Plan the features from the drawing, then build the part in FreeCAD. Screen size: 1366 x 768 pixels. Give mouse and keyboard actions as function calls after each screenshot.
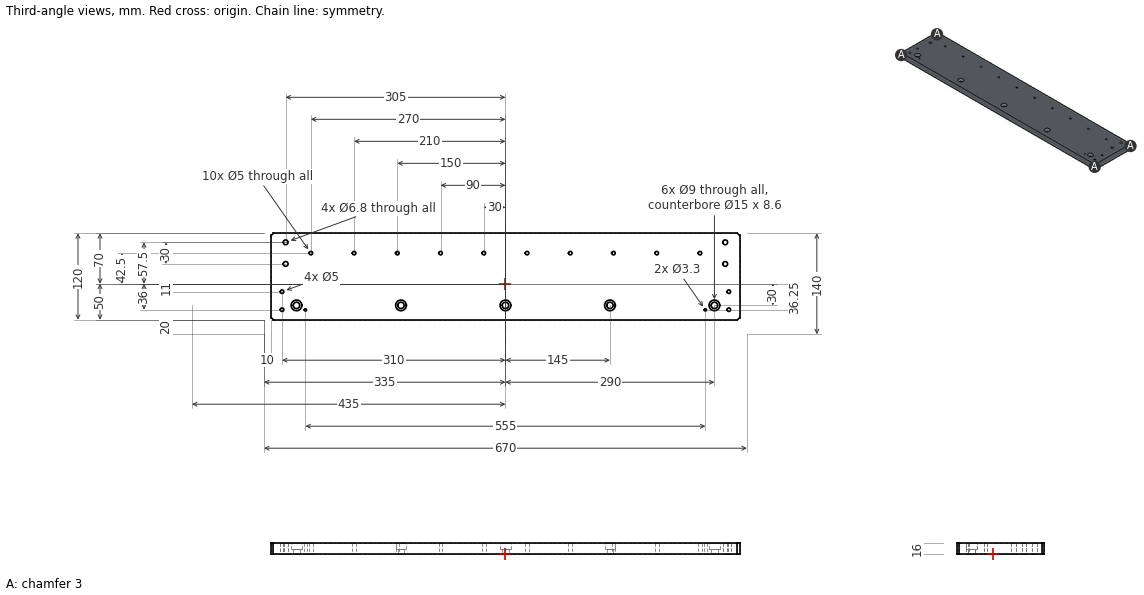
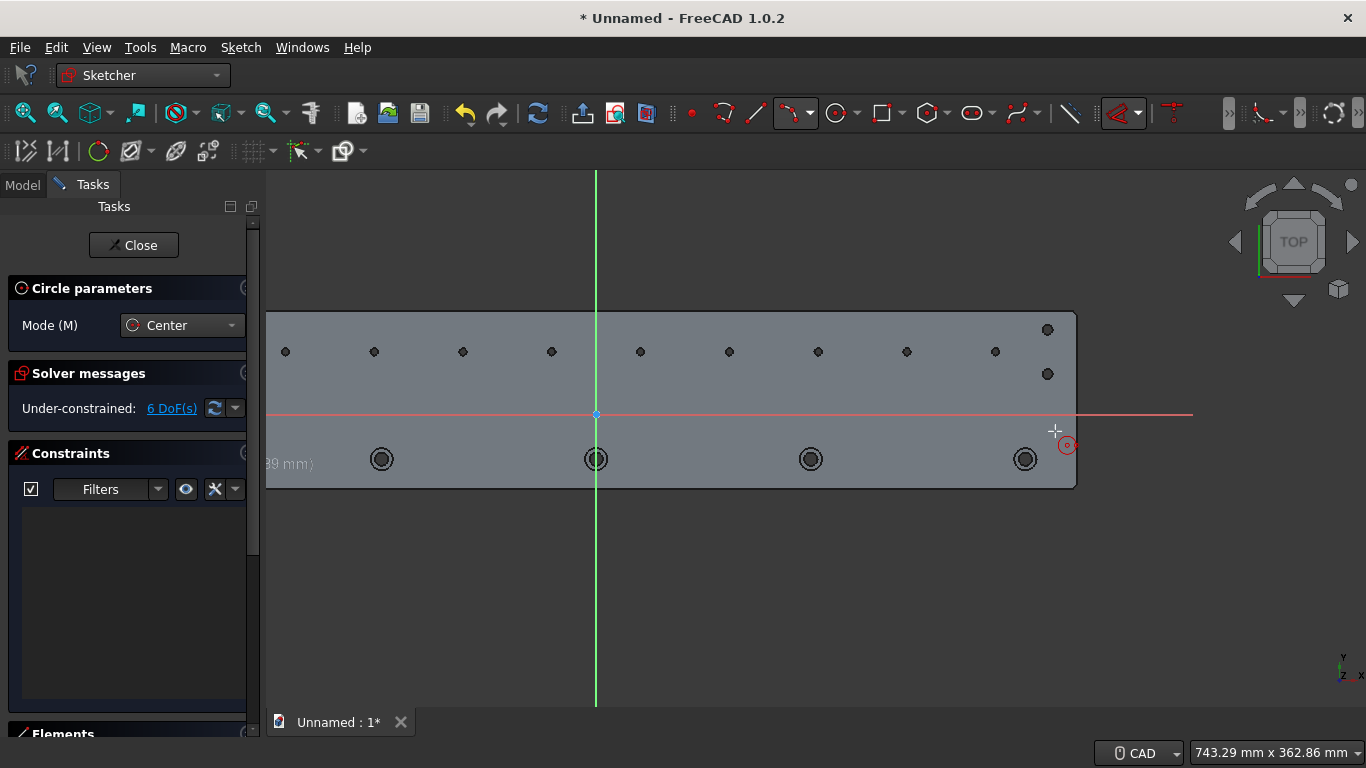
click(1055, 431)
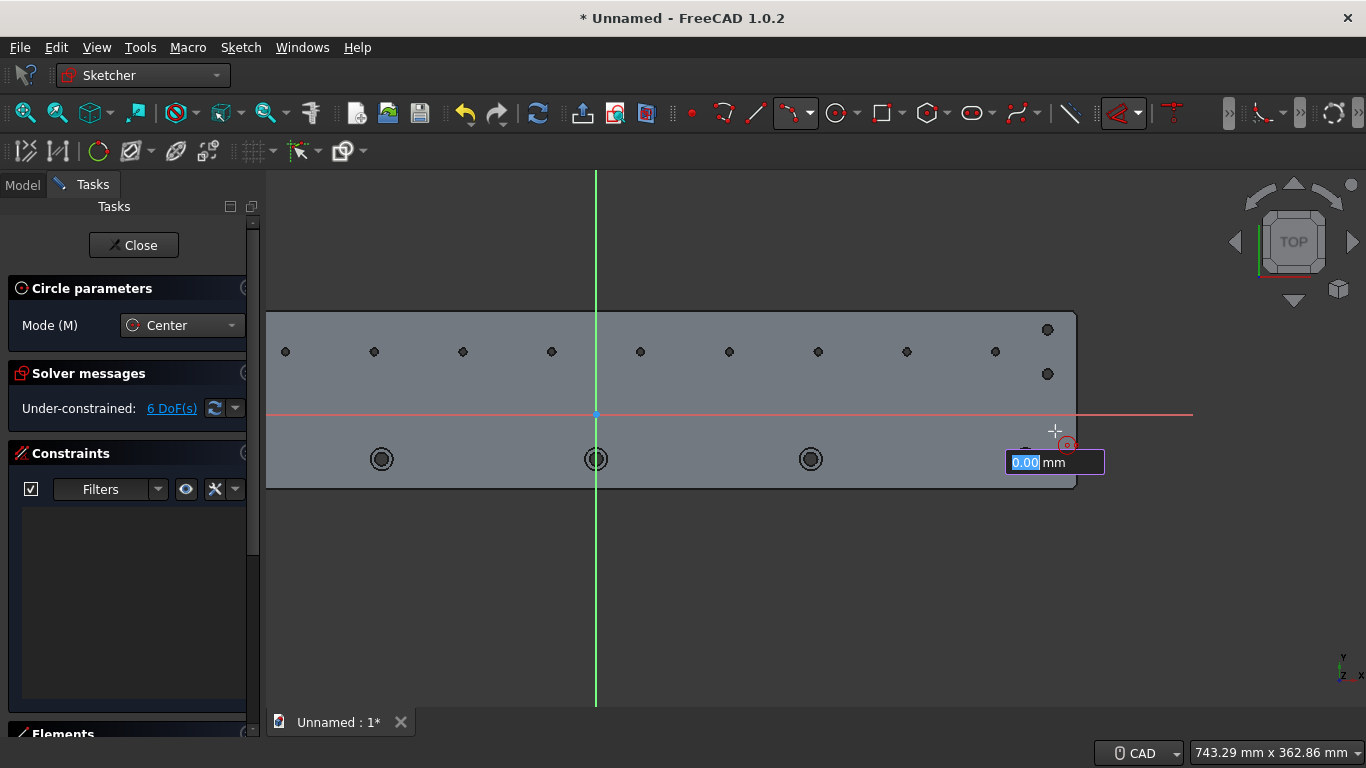
scroll(1058, 434, up, 8)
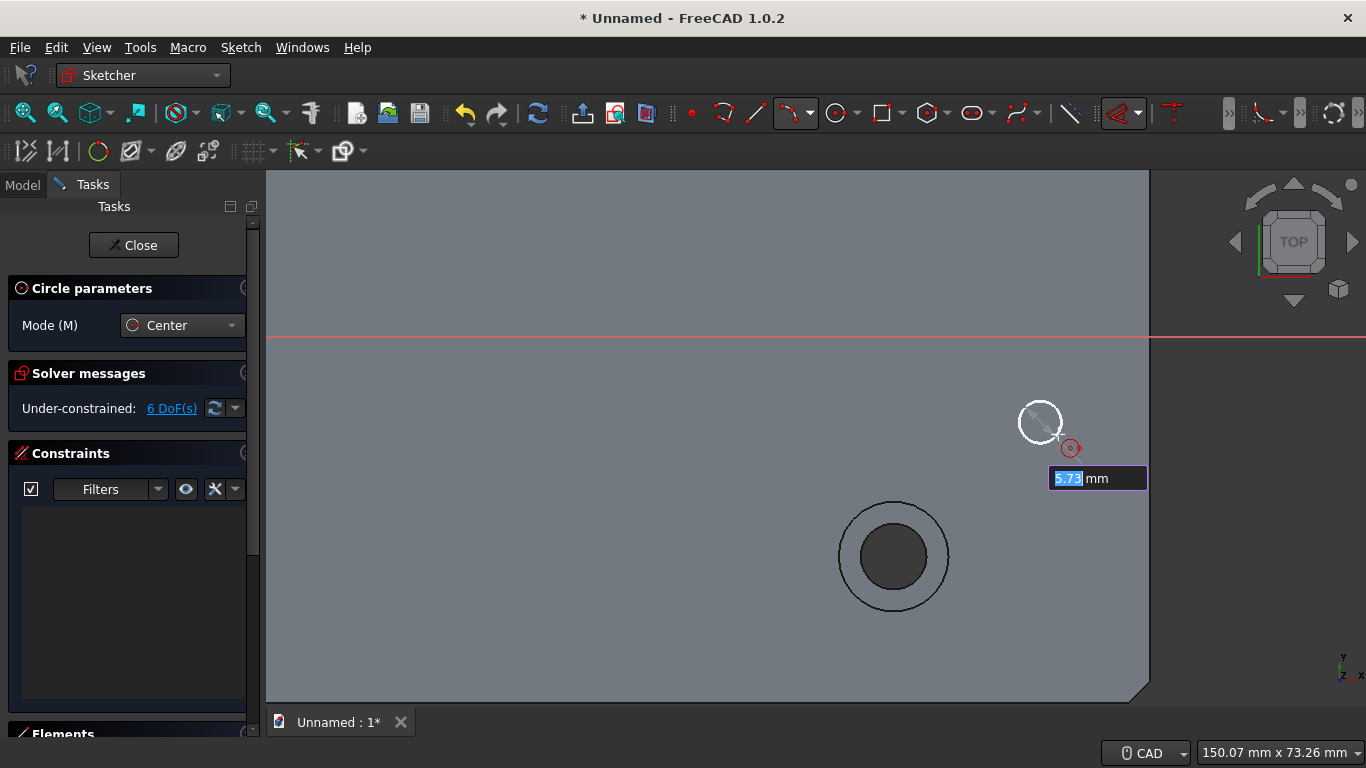
click(1053, 430)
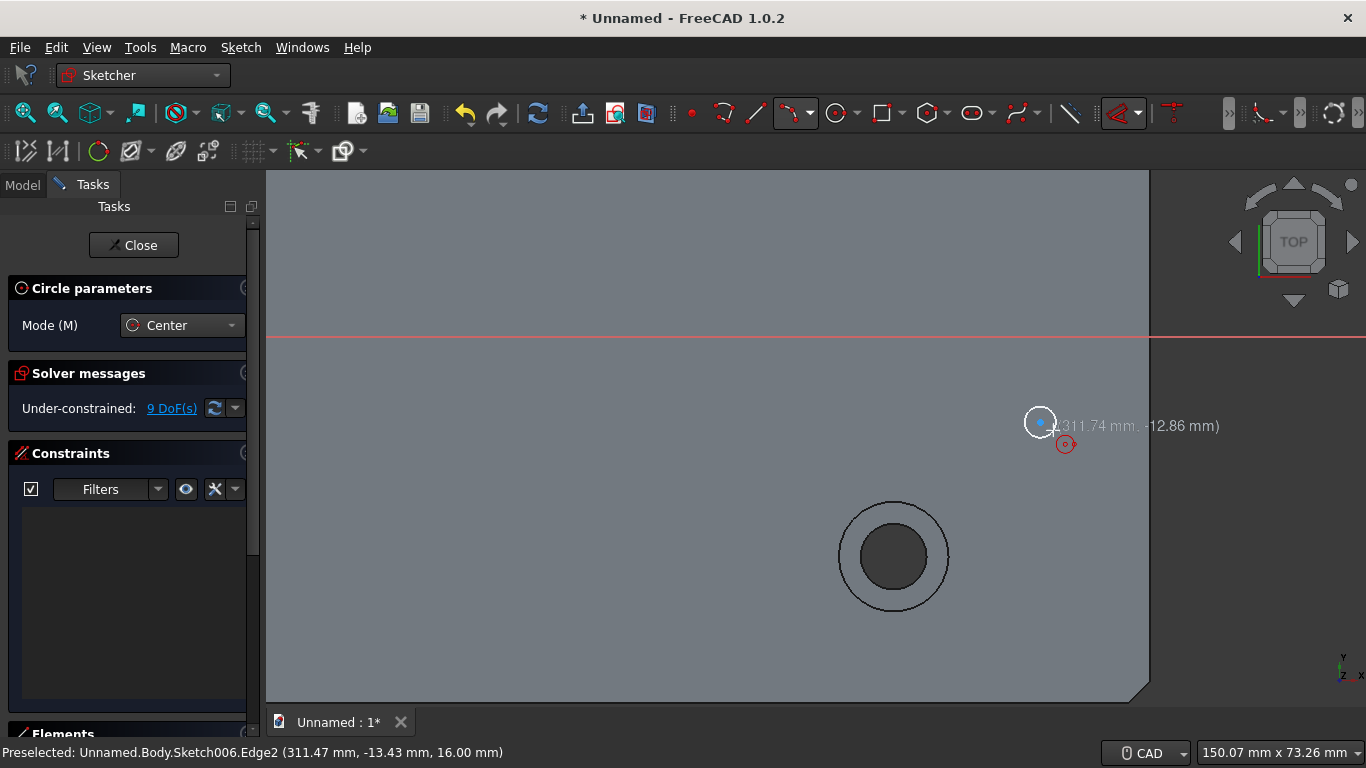
scroll(1040, 601, up, 2)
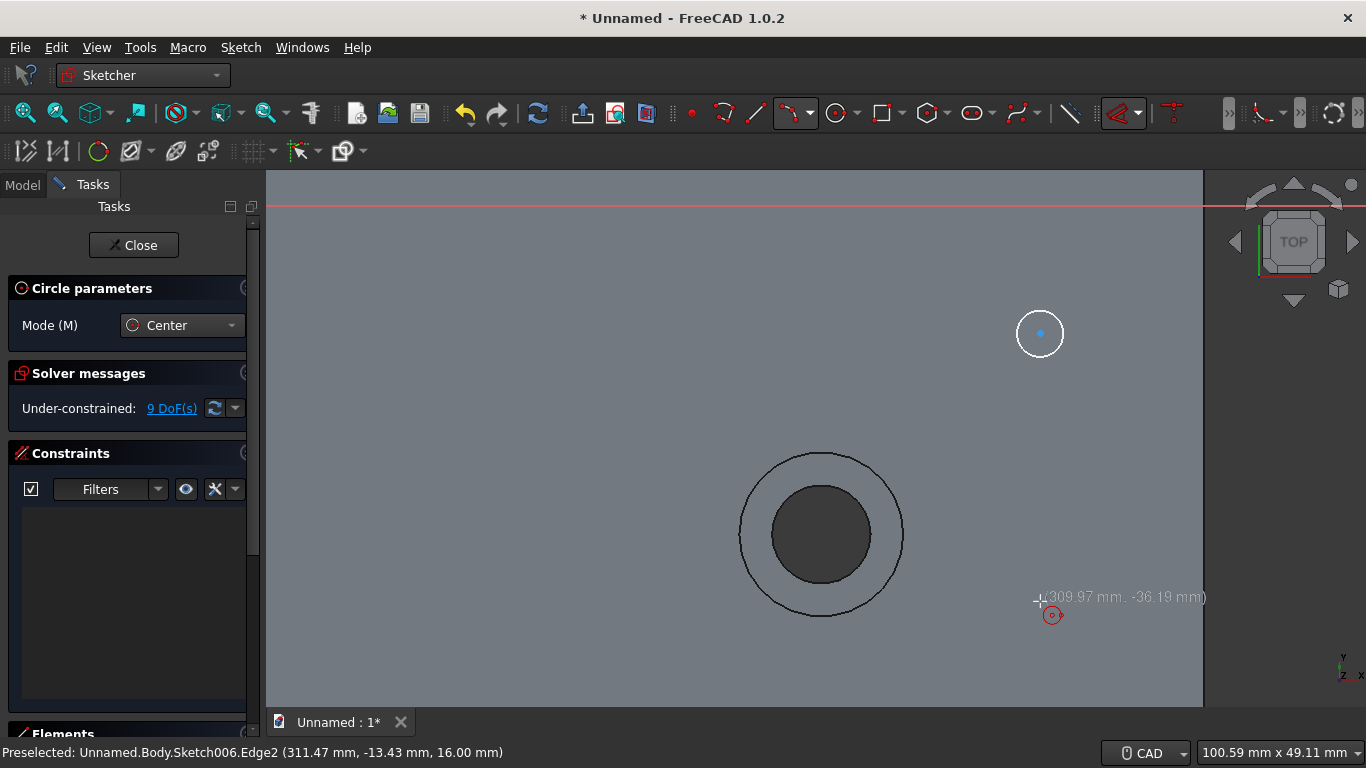
scroll(1057, 441, down, 12)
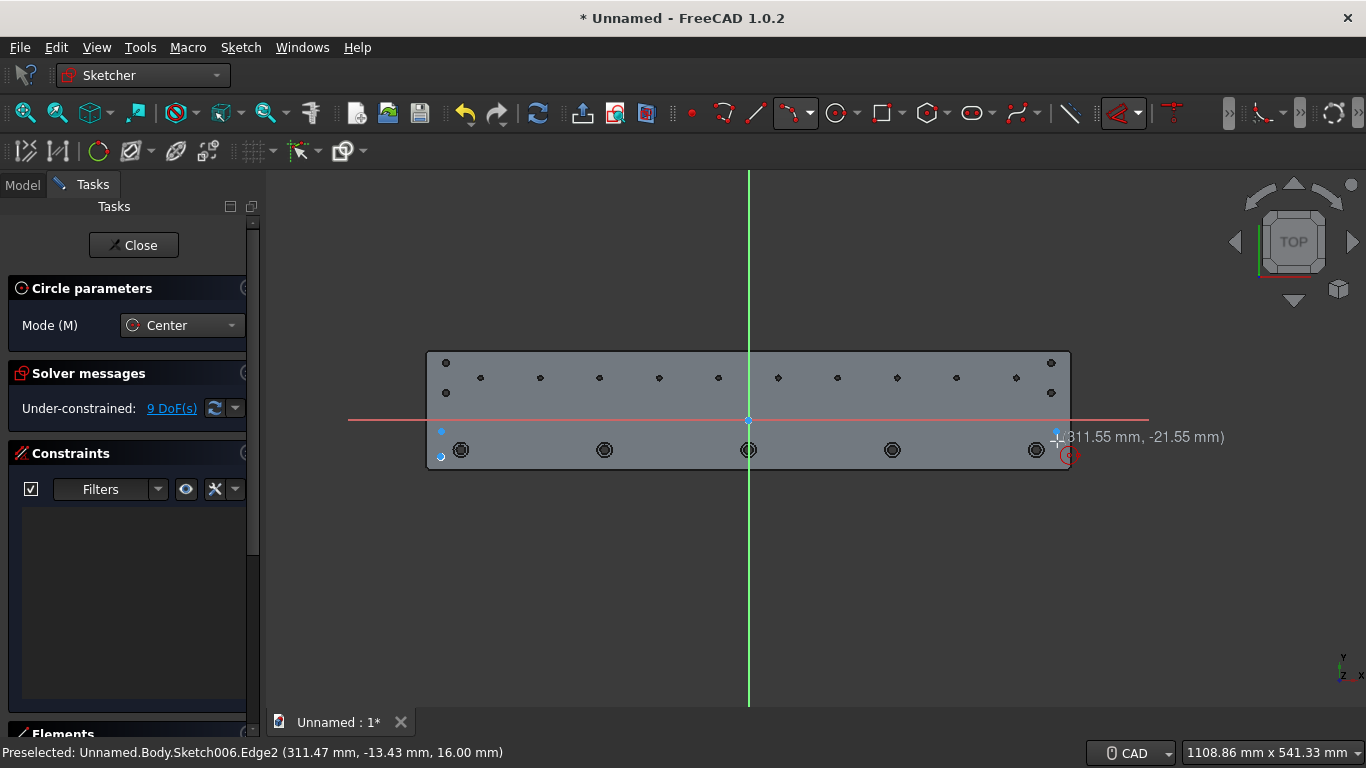
click(1056, 456)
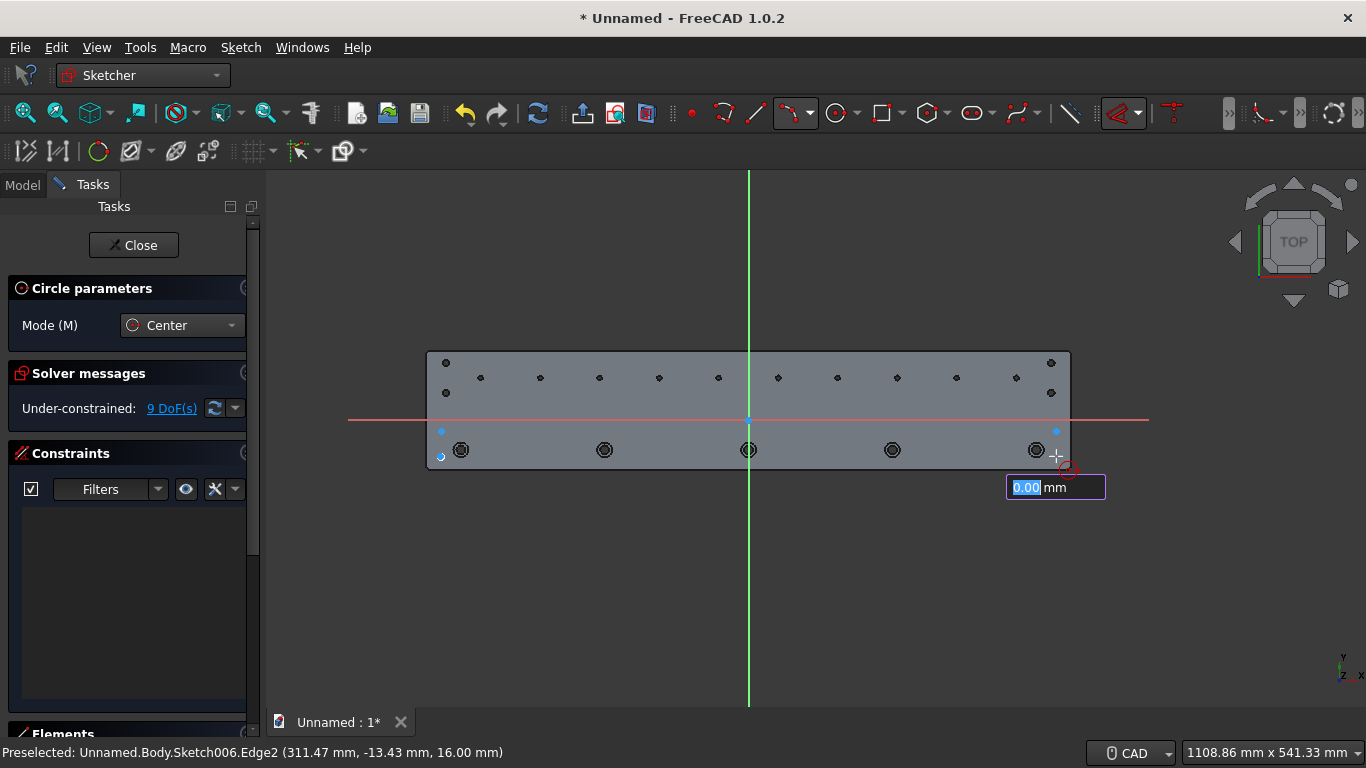
scroll(1058, 454, up, 10)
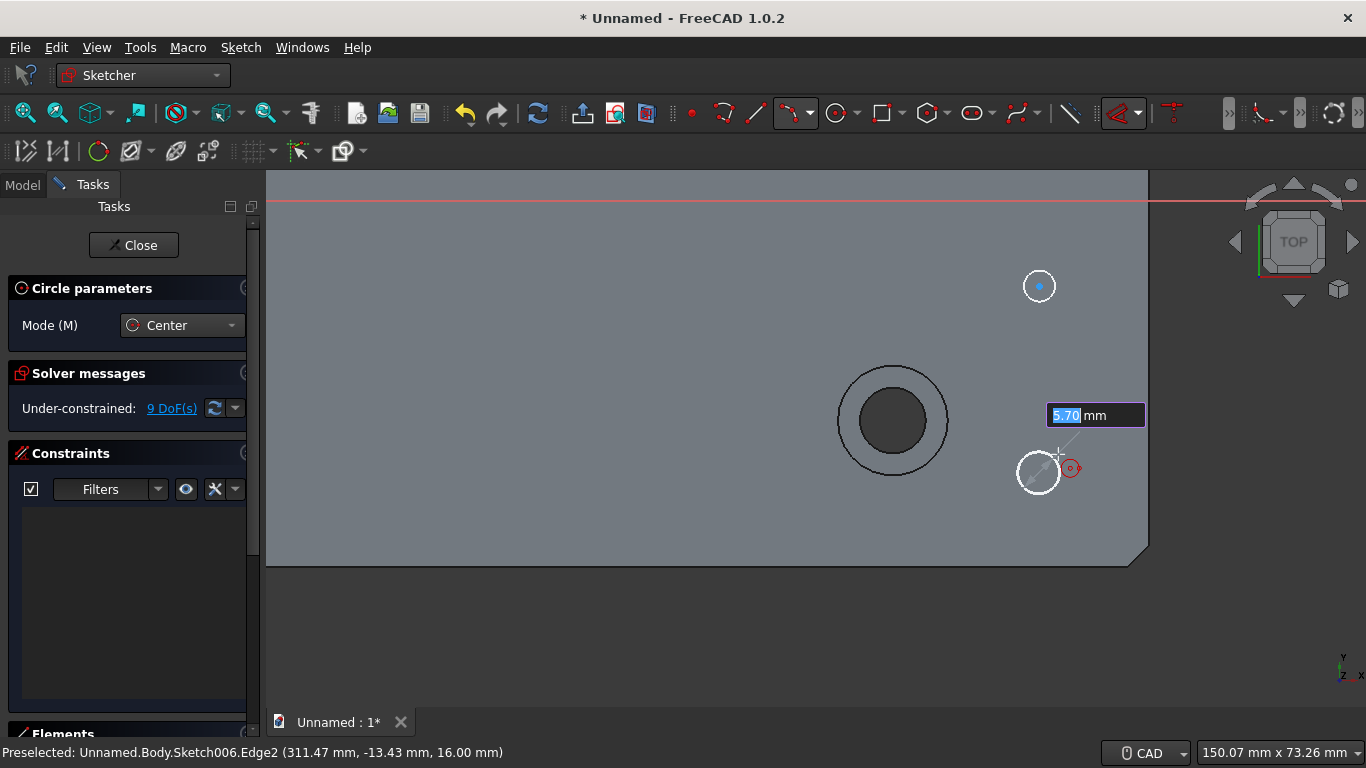
click(1052, 452)
key(Escape)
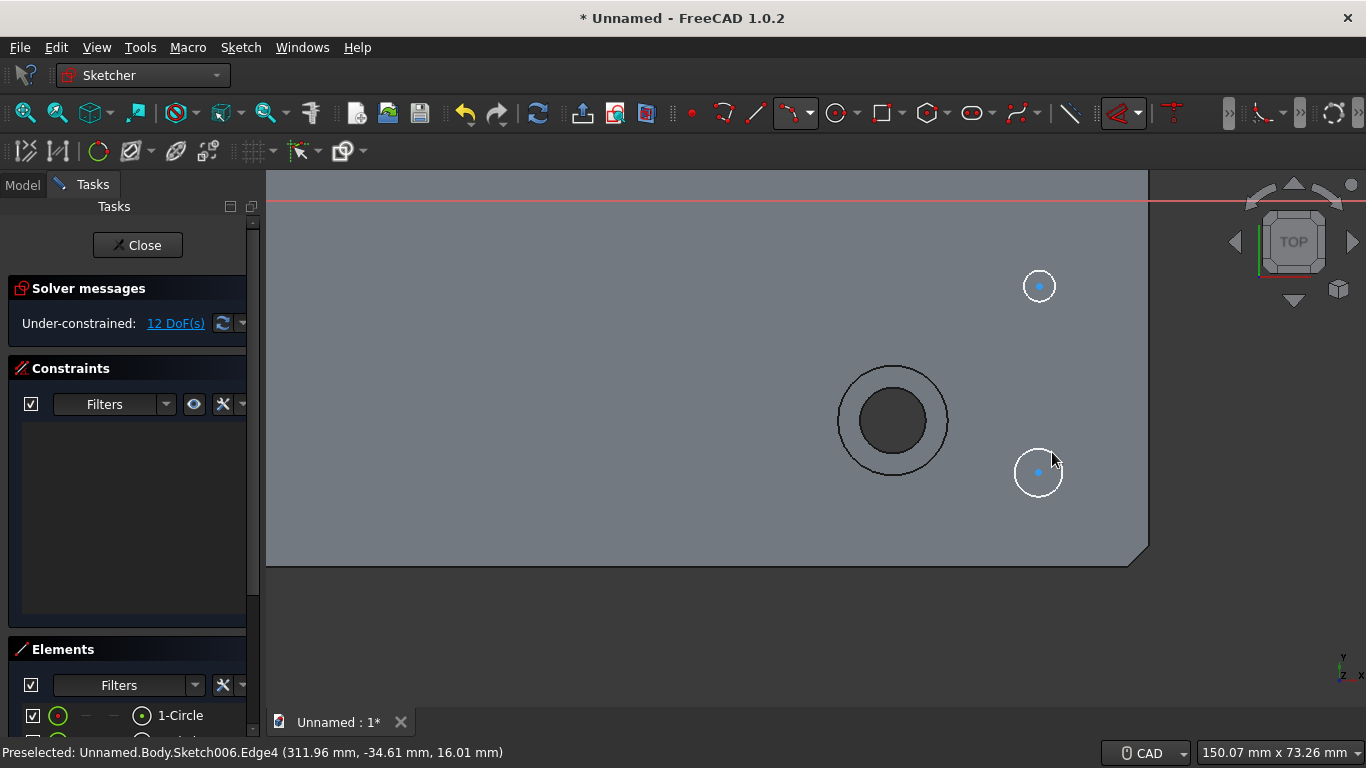
scroll(1057, 454, down, 10)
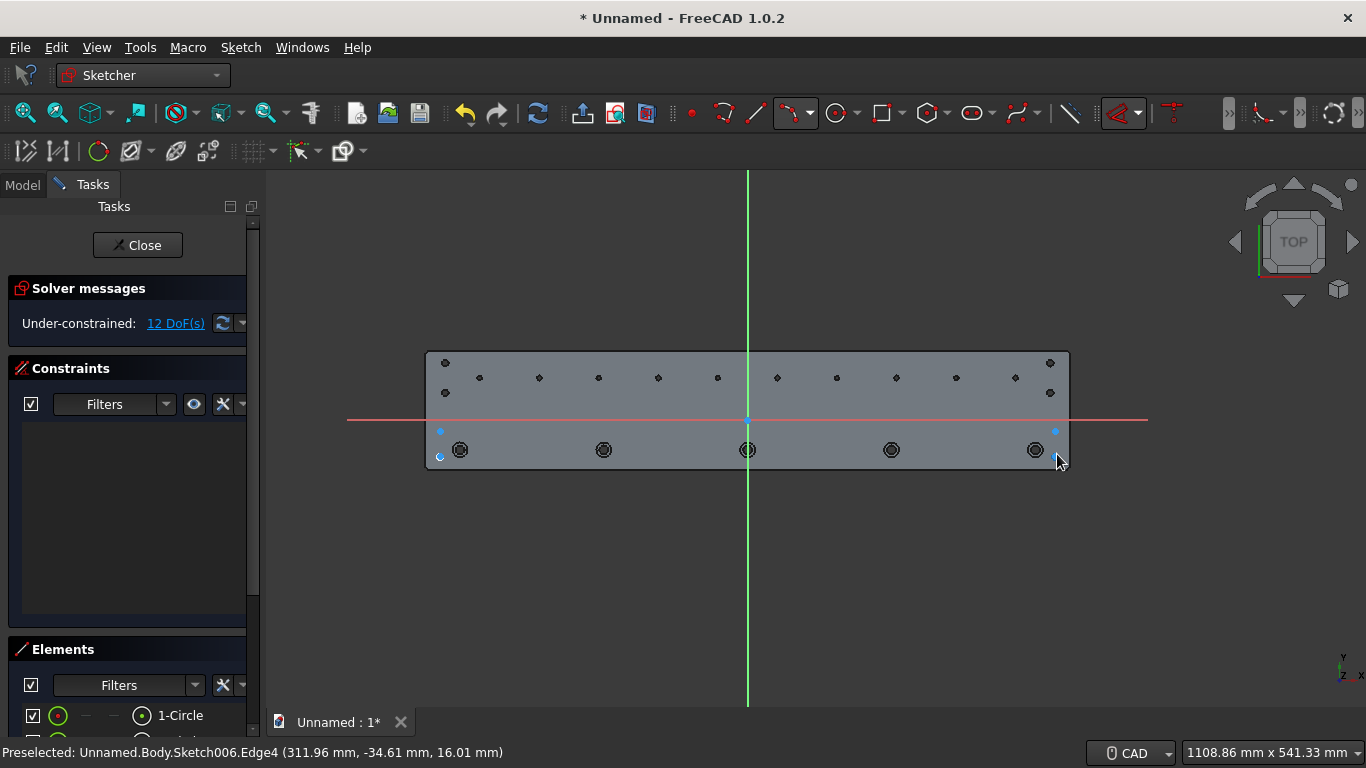
scroll(442, 430, up, 10)